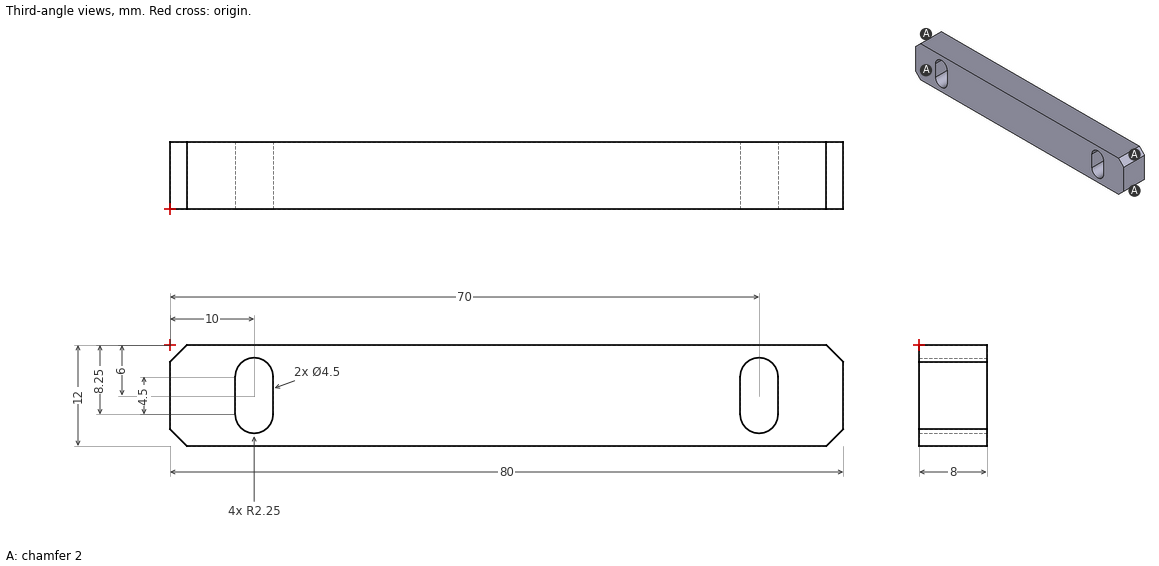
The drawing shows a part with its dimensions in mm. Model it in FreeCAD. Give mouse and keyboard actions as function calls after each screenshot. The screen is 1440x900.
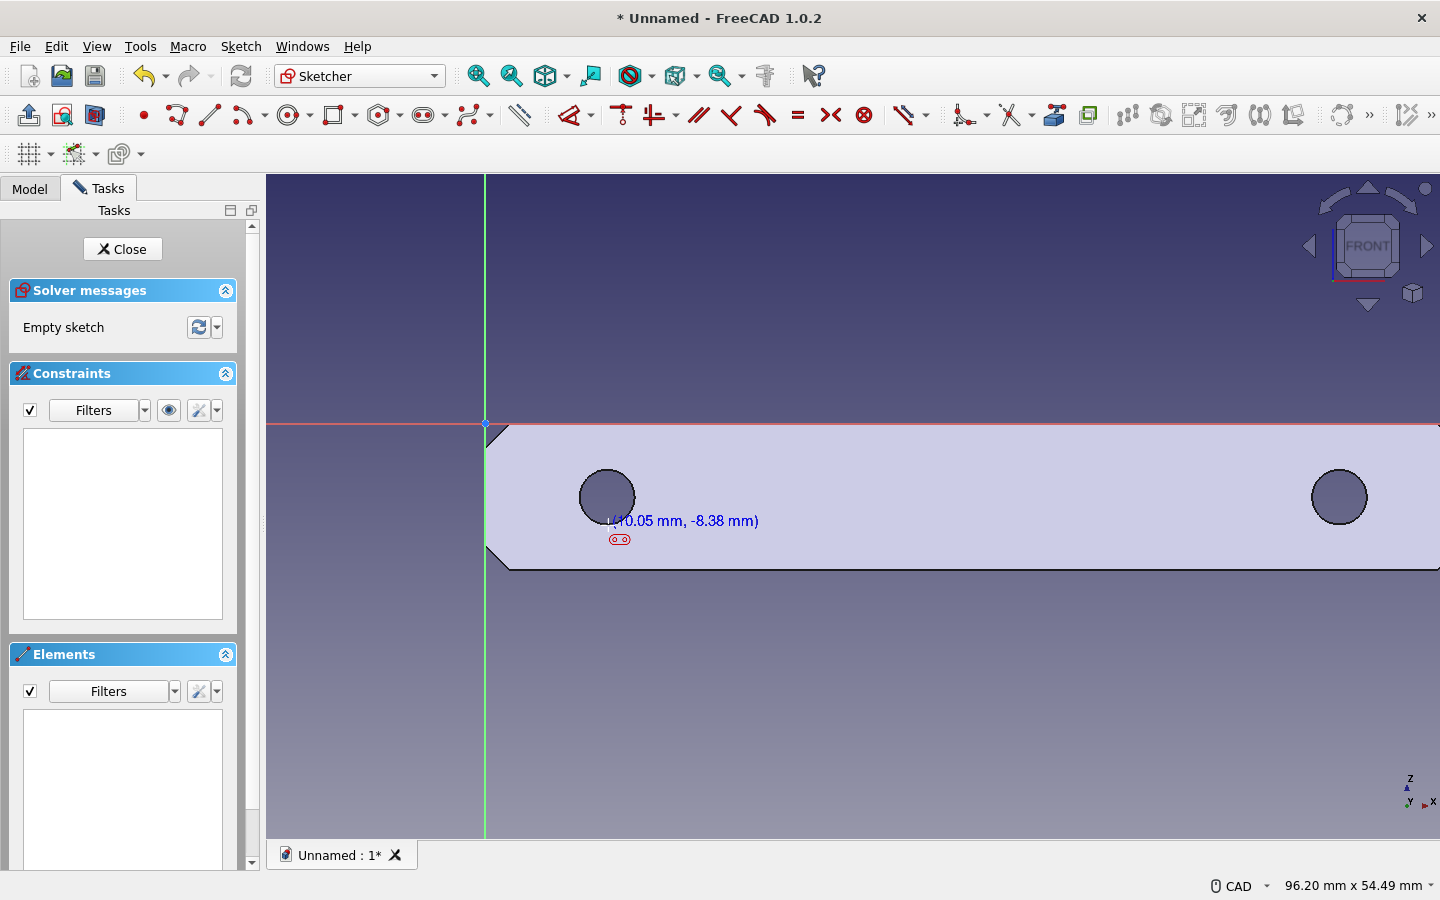
click(607, 525)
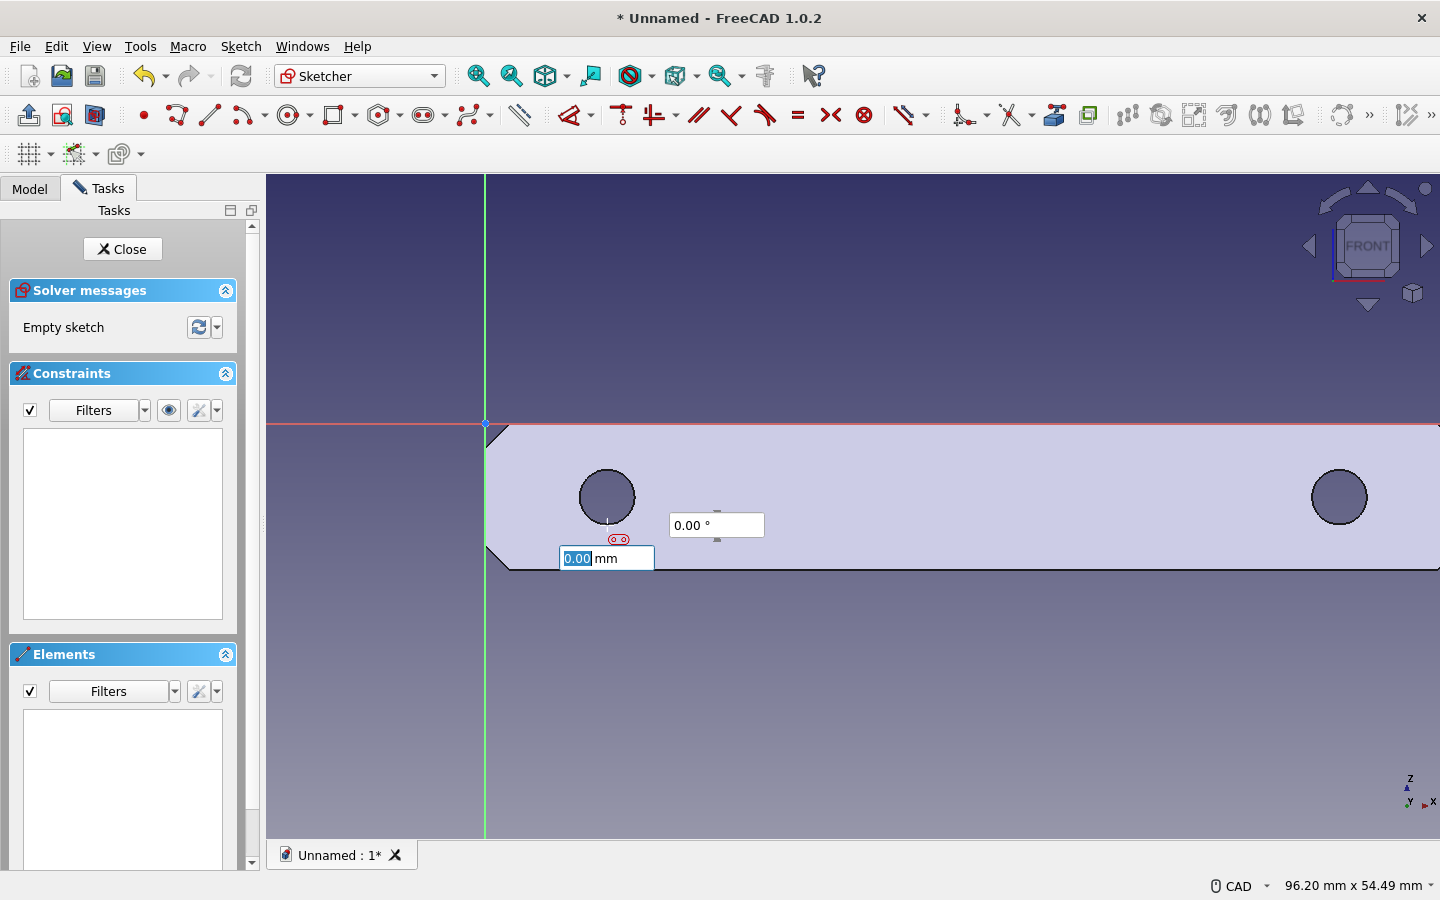
click(607, 470)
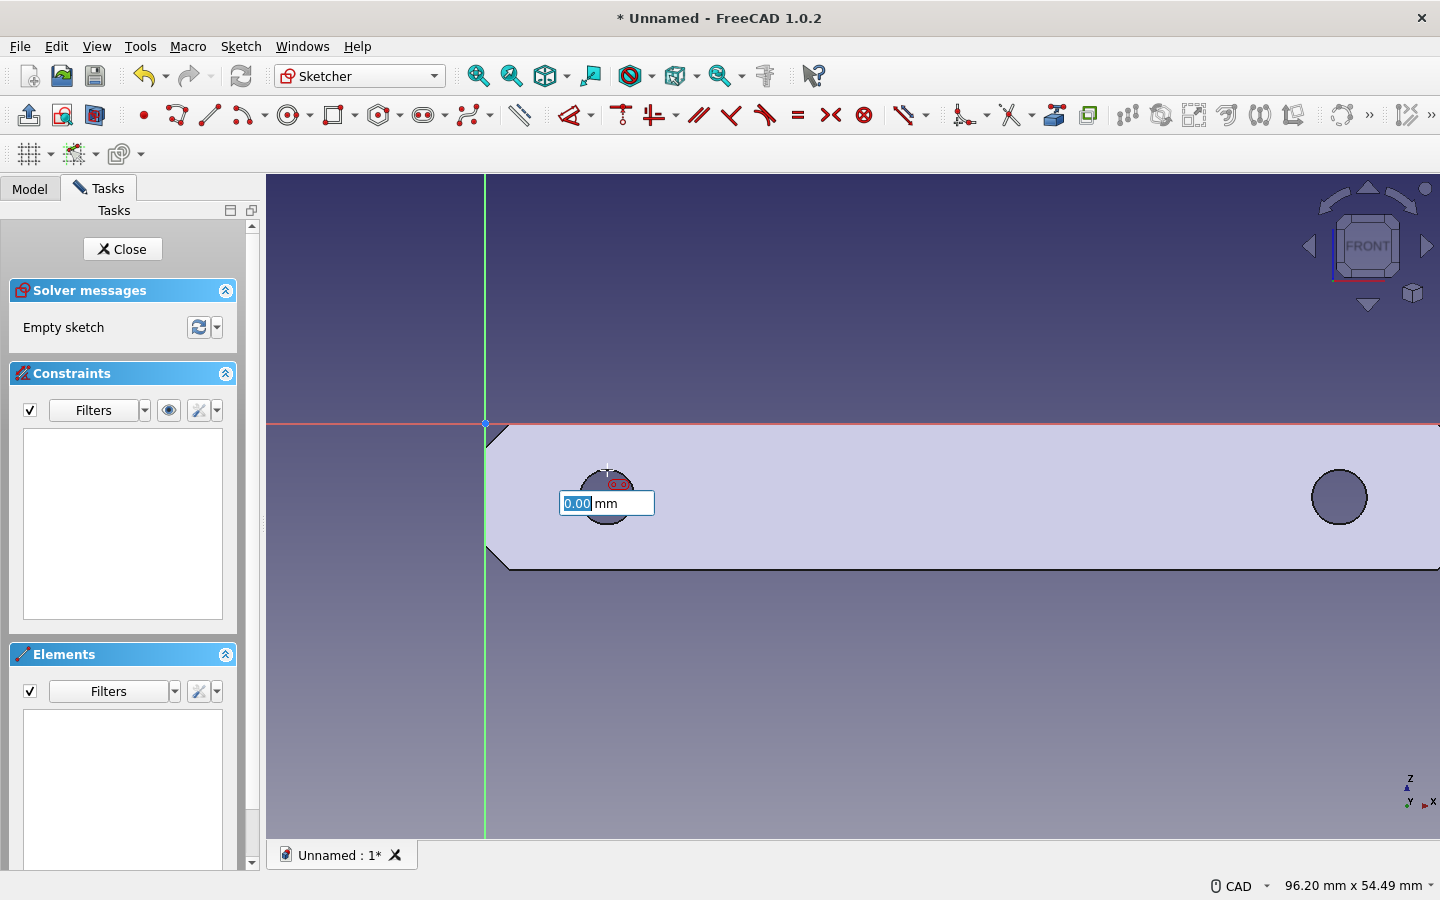
click(580, 497)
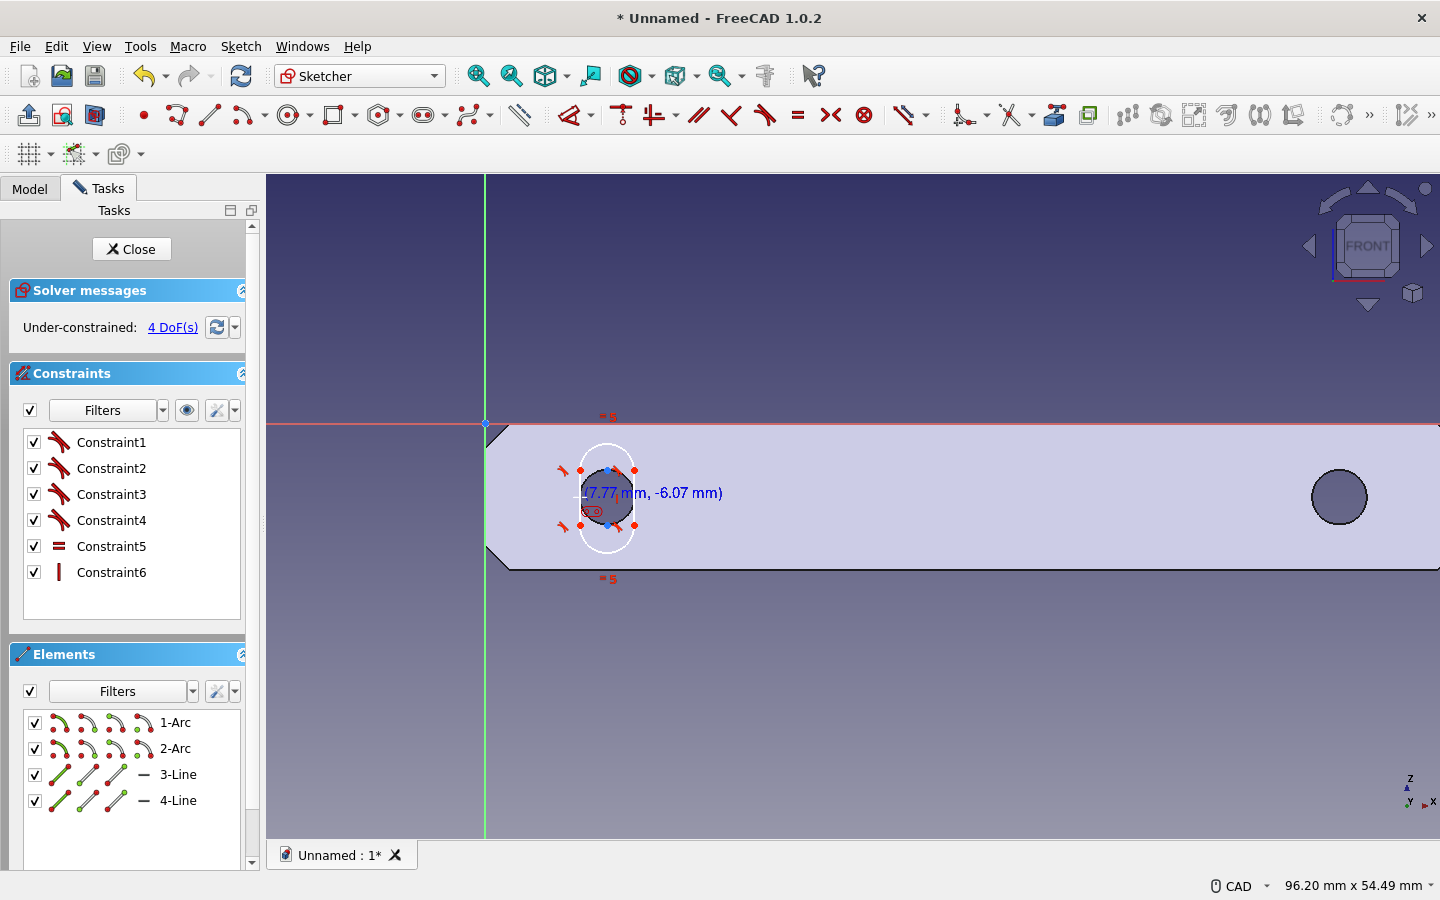
scroll(294, 590, down, 1)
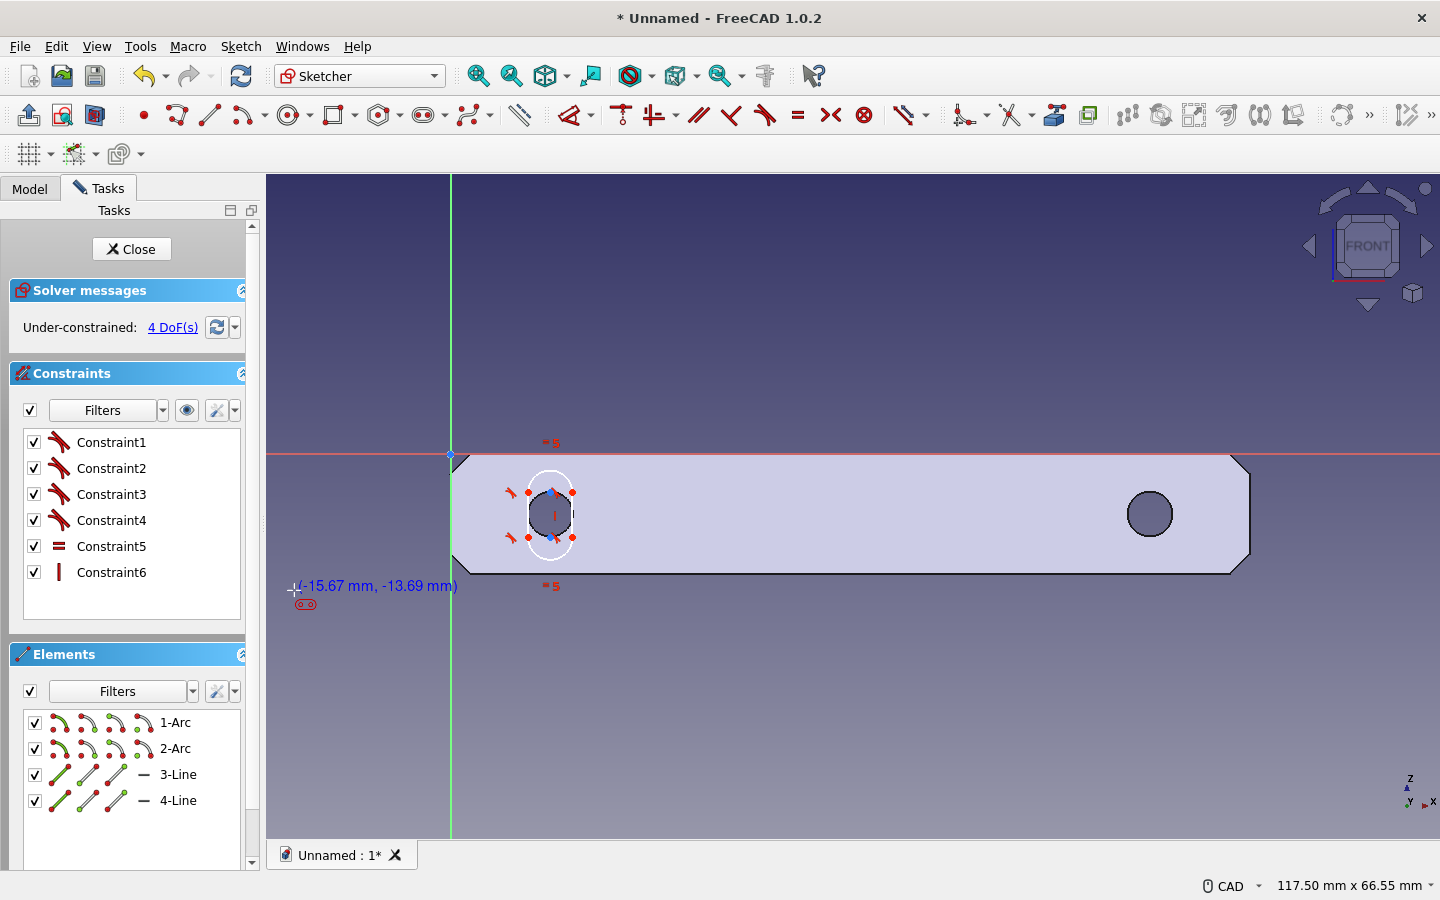
click(1150, 537)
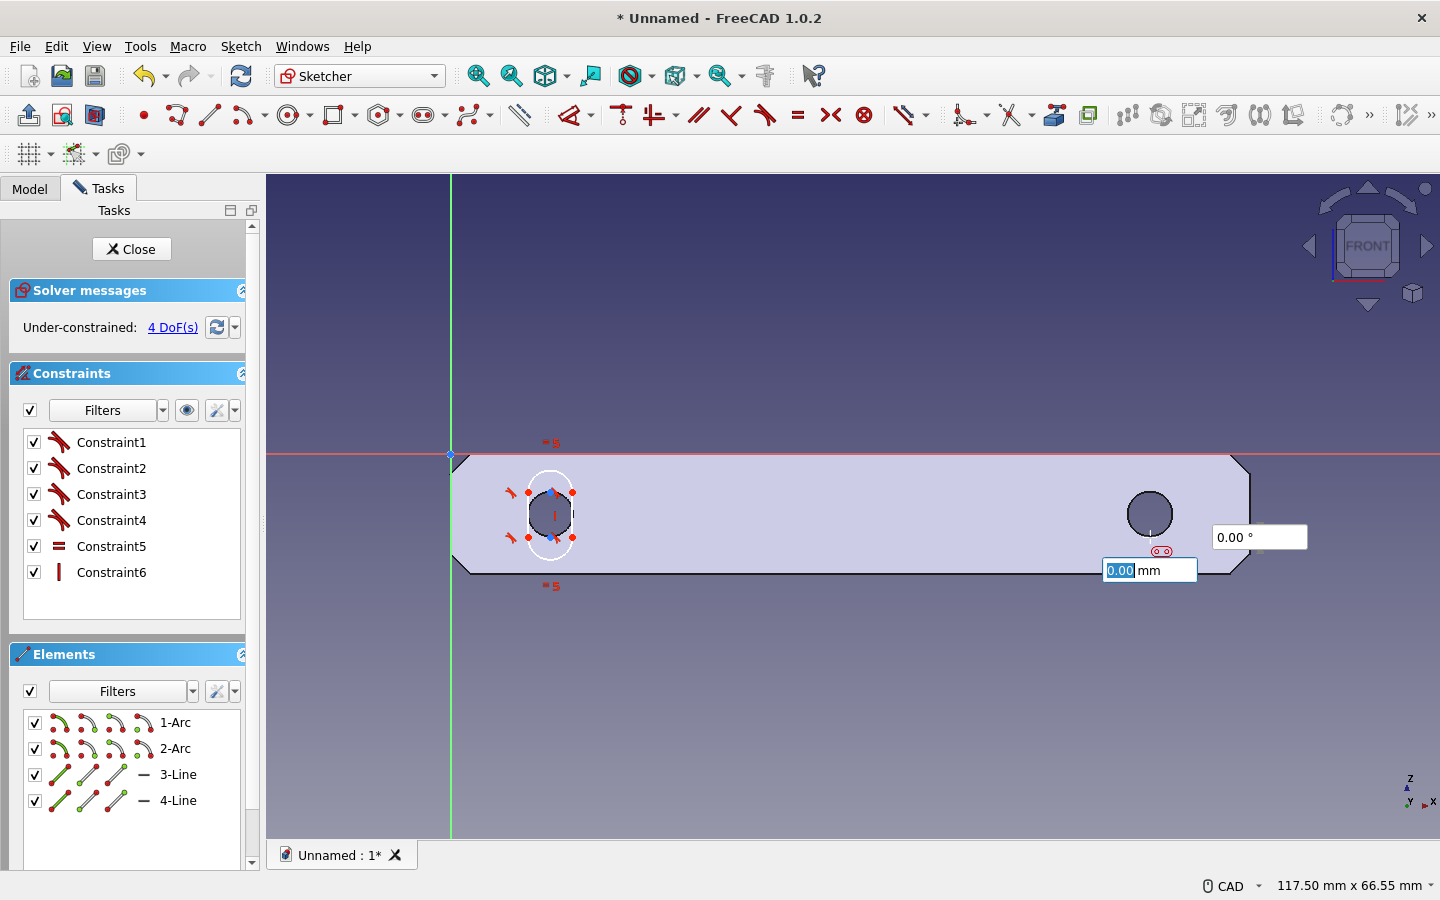
click(1150, 492)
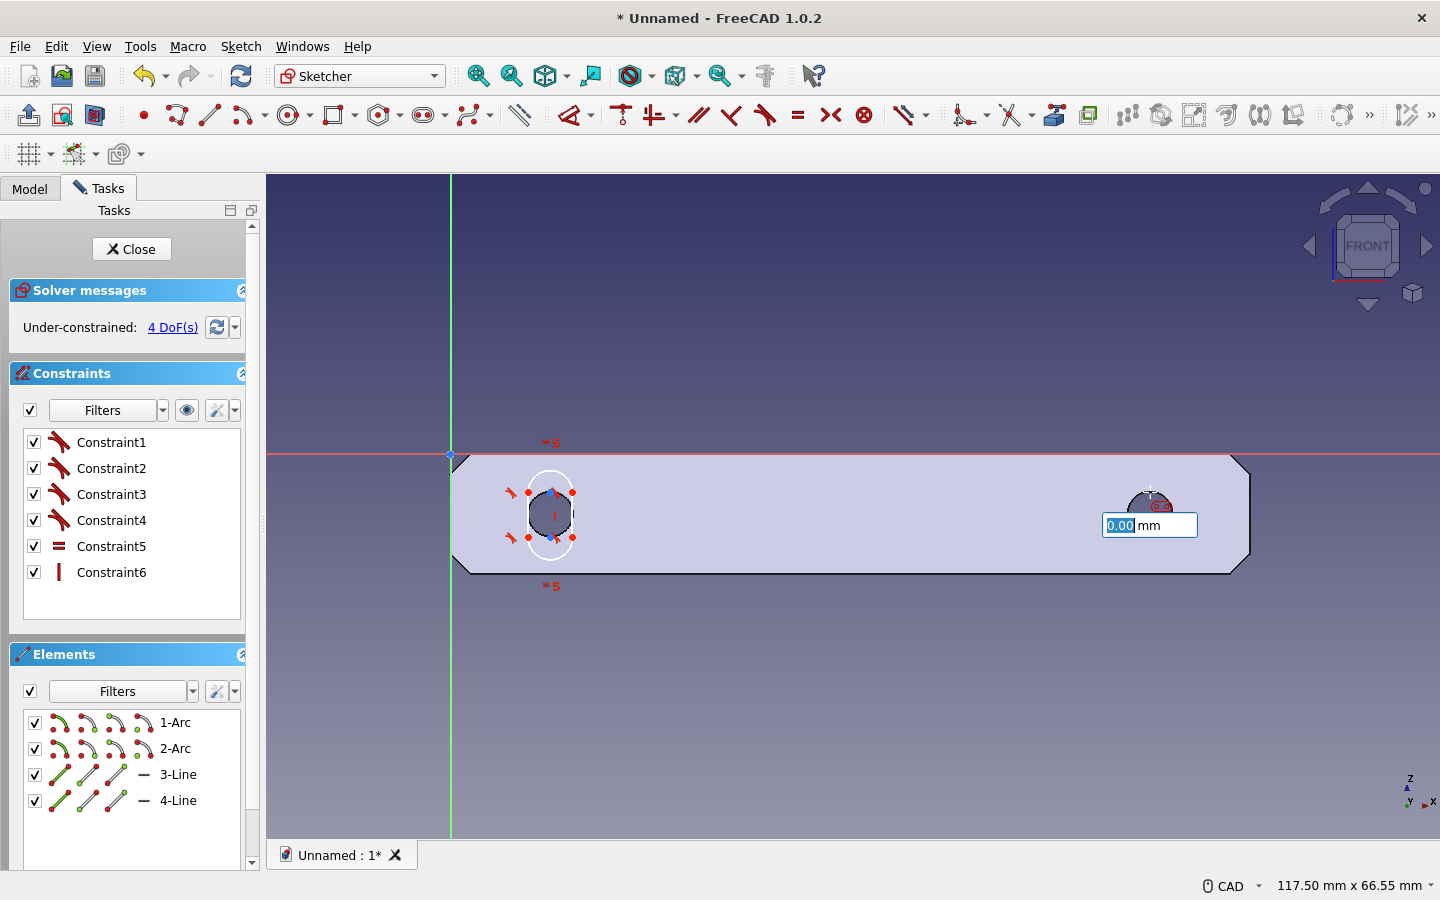
click(1172, 514)
key(Escape)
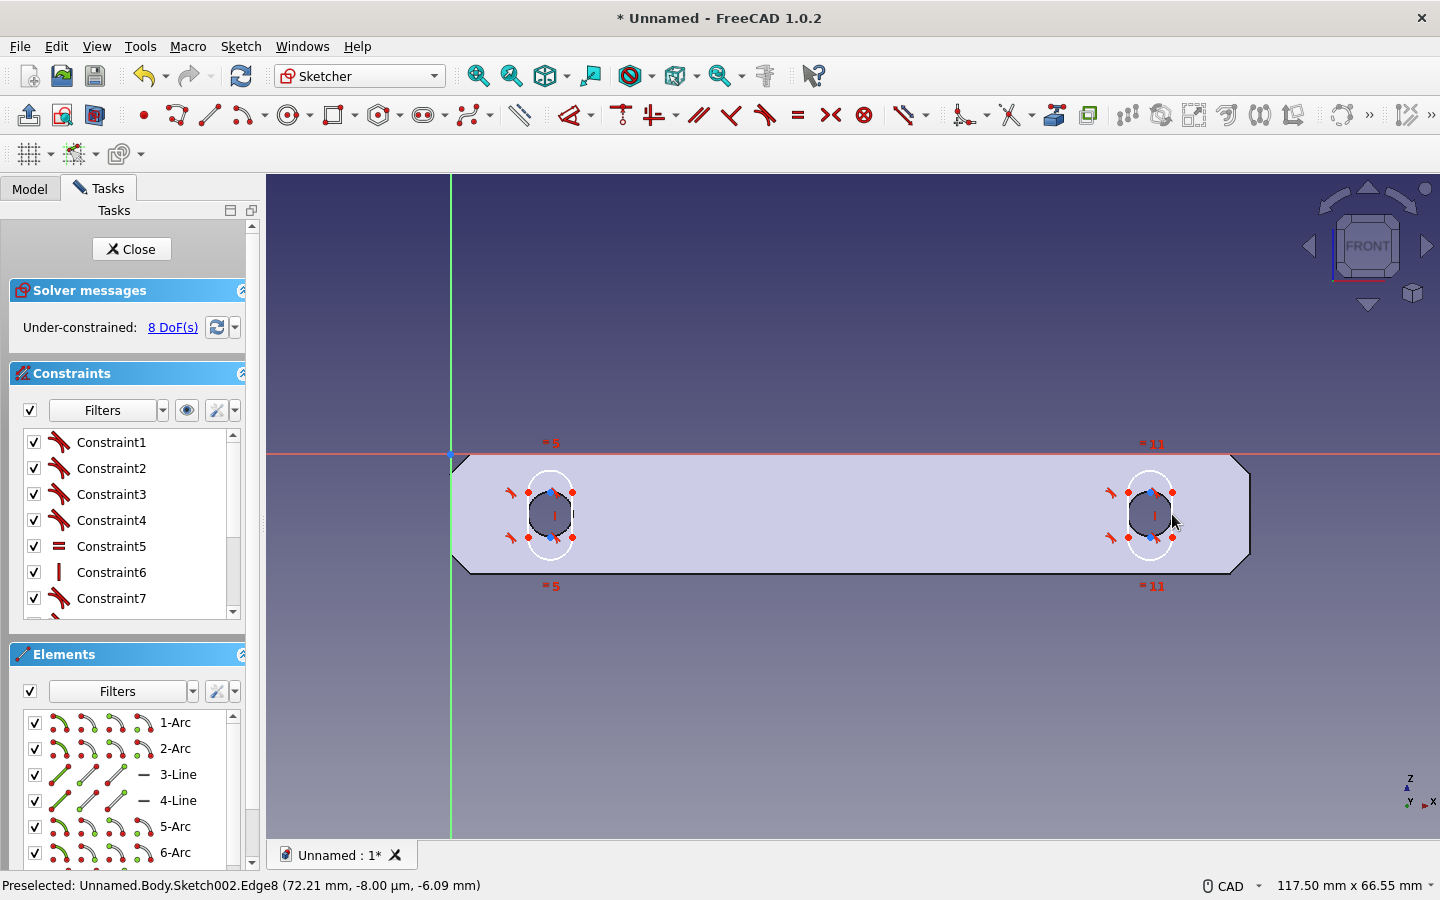
click(537, 556)